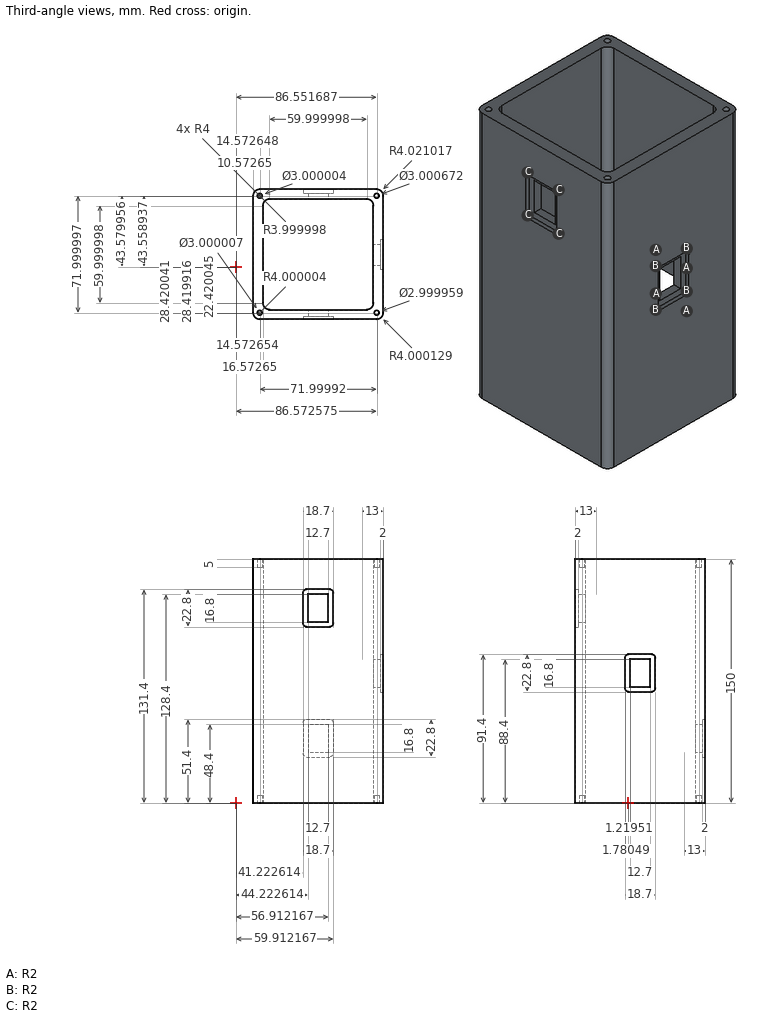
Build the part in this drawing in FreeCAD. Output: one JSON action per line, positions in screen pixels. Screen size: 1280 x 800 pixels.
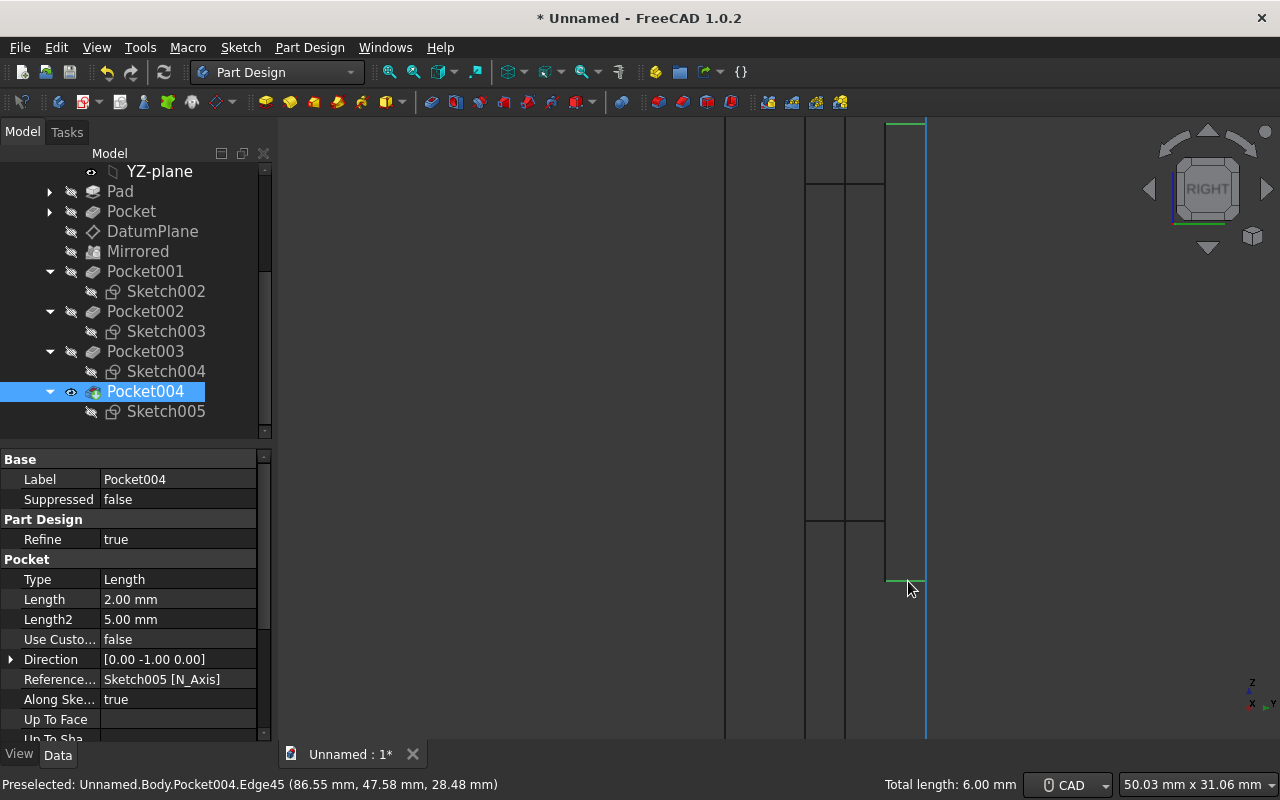
{"action": "left_click", "coordinate": [390, 72]}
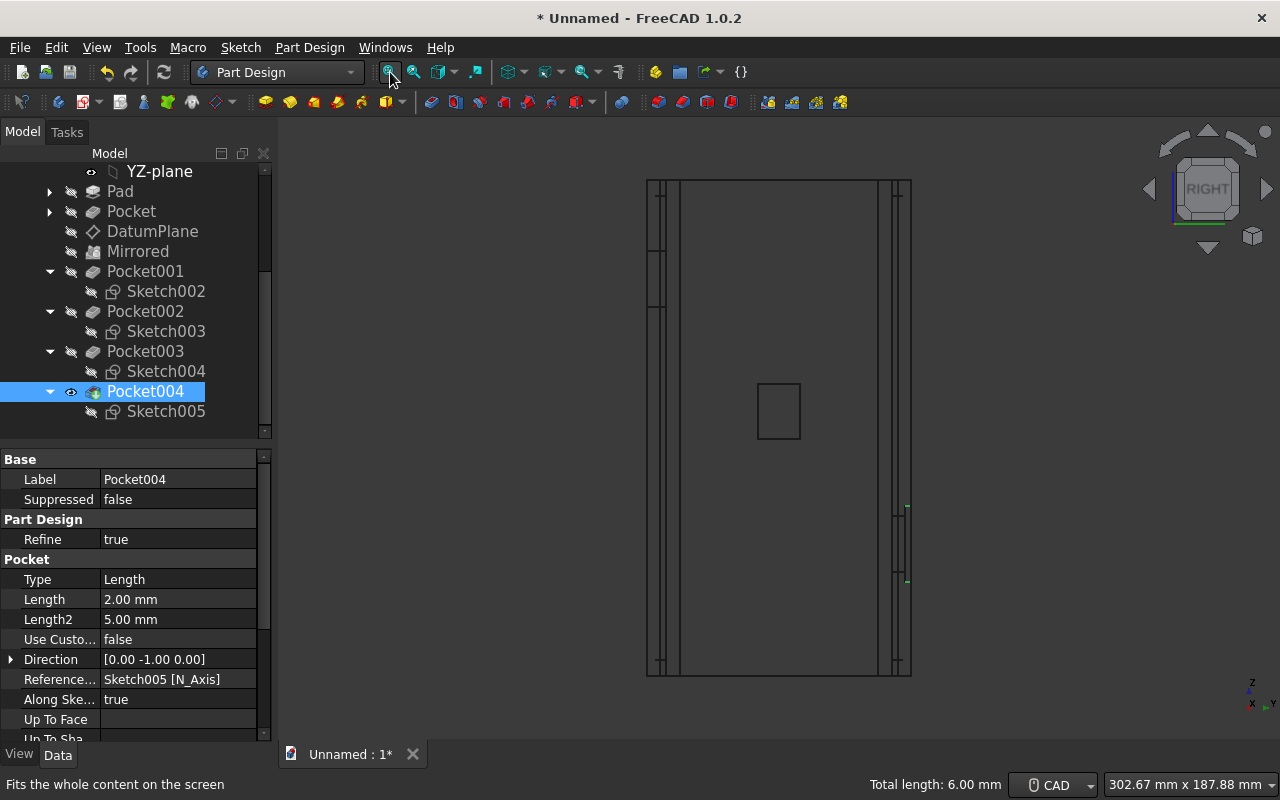
{"action": "key", "text": "5"}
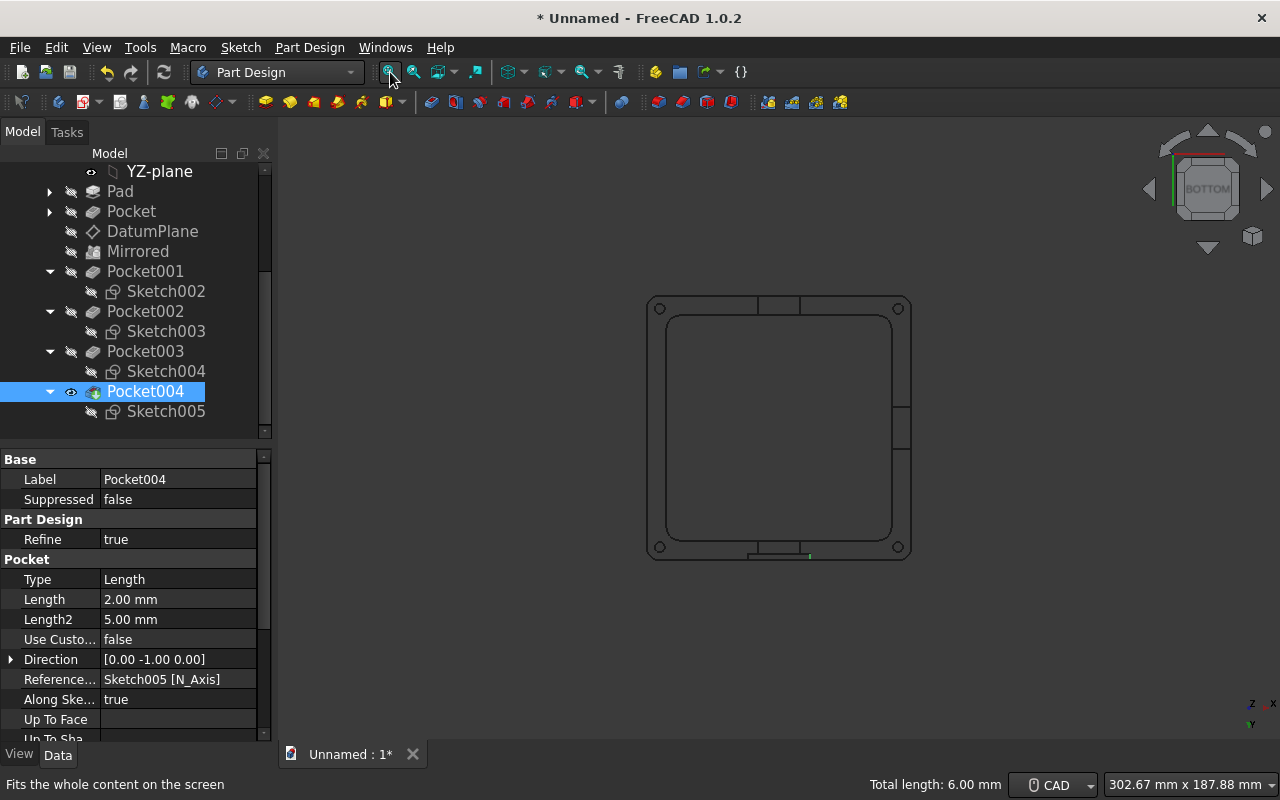
{"action": "left_click", "coordinate": [390, 72]}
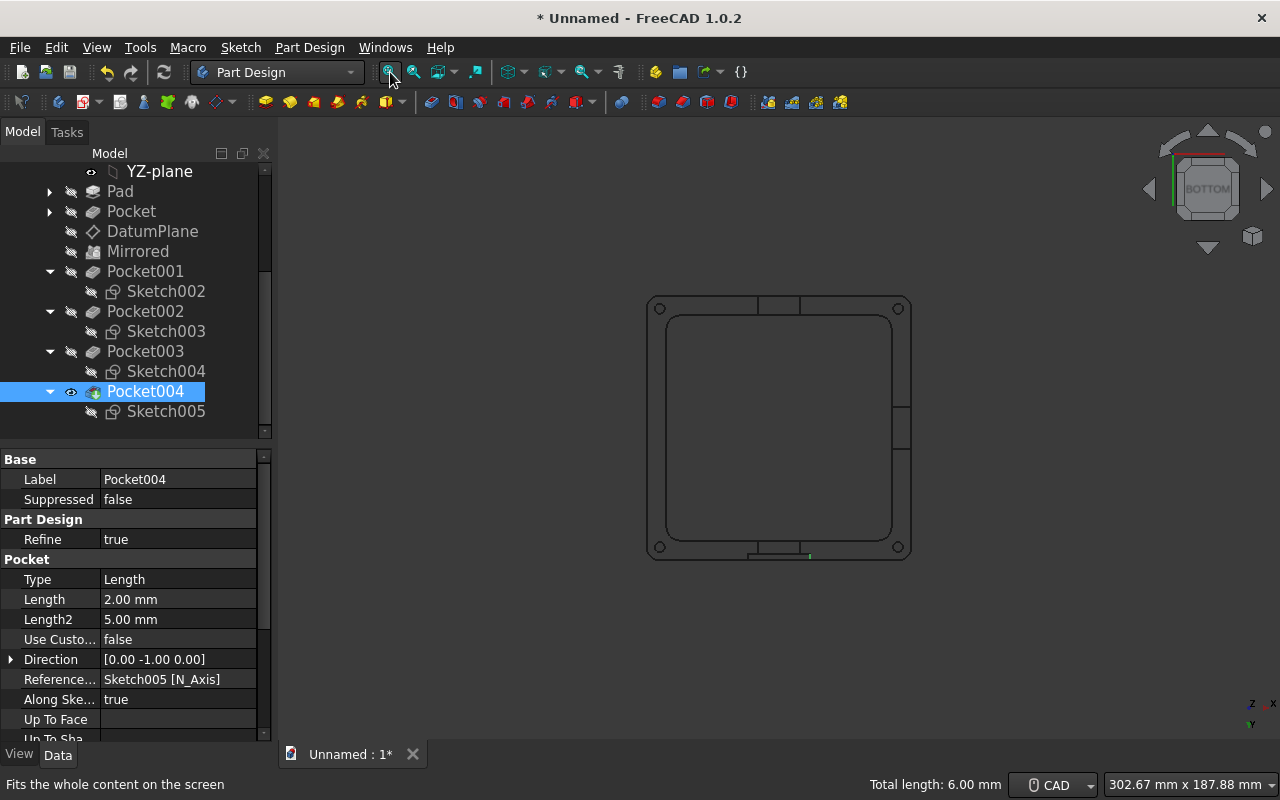
{"action": "scroll", "coordinate": [748, 556], "scroll_direction": "up", "scroll_amount": 9}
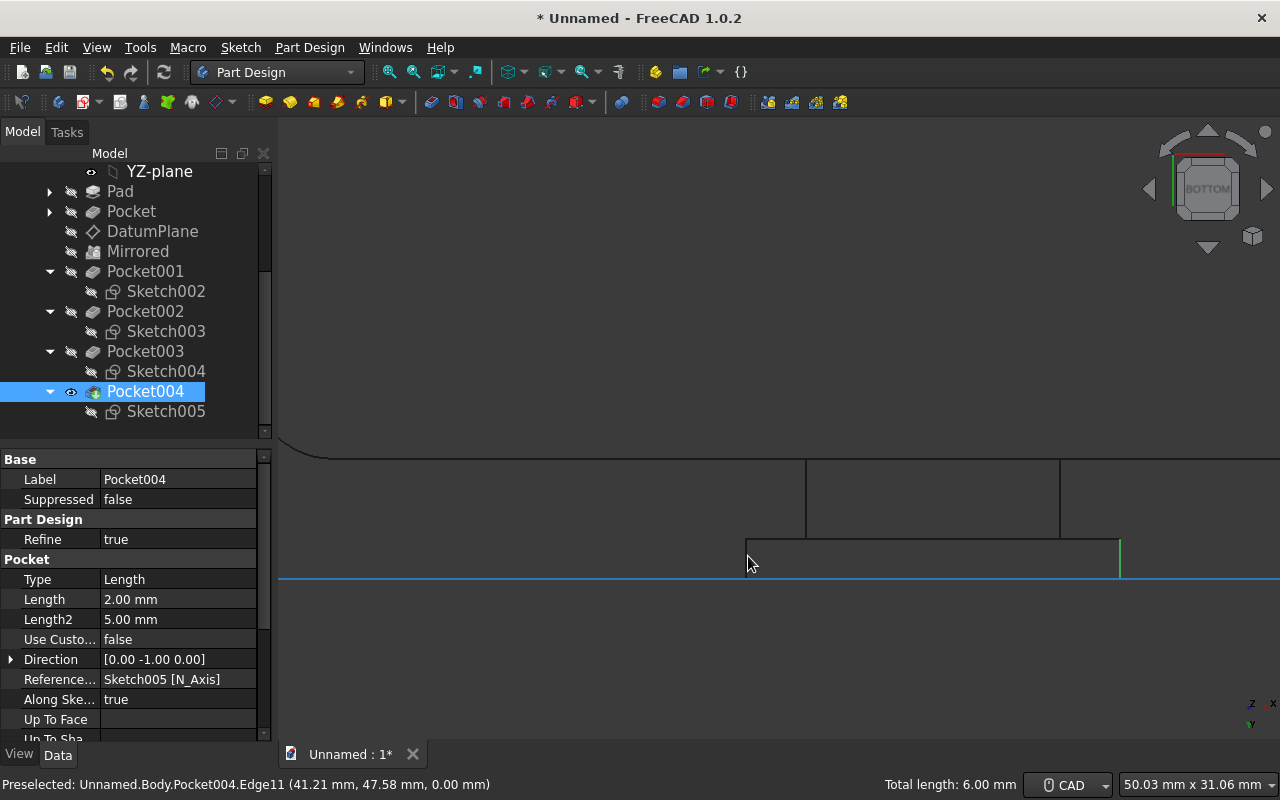
{"action": "left_click", "coordinate": [746, 558], "text": "ctrl"}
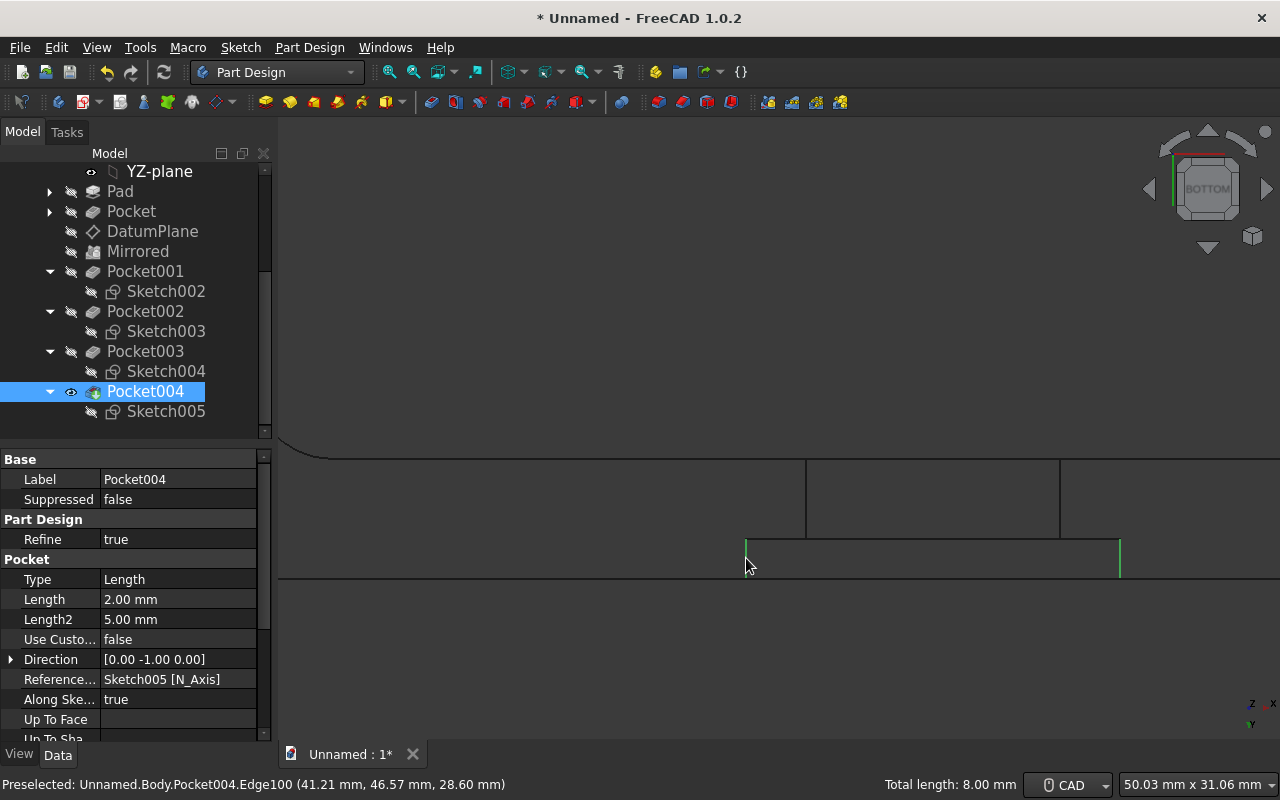
{"action": "key", "text": "v 1"}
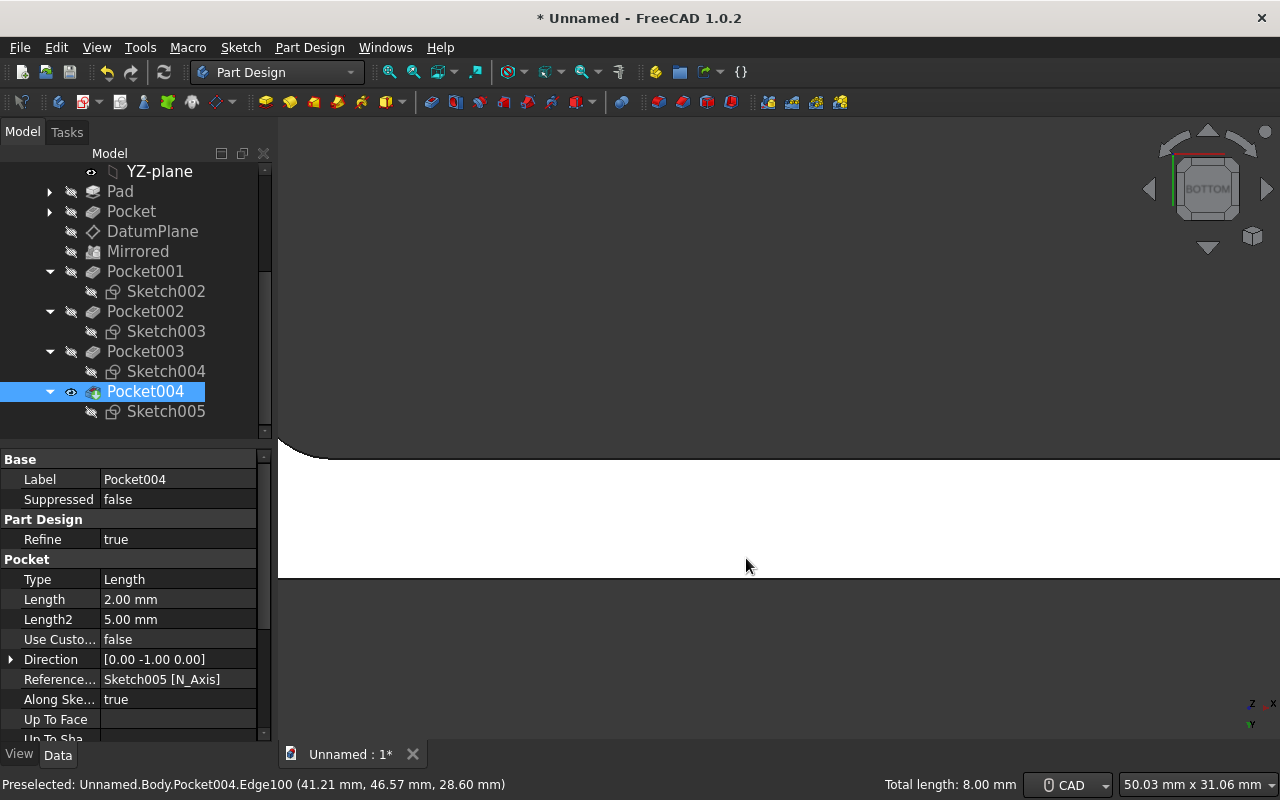
{"action": "left_click", "coordinate": [660, 102]}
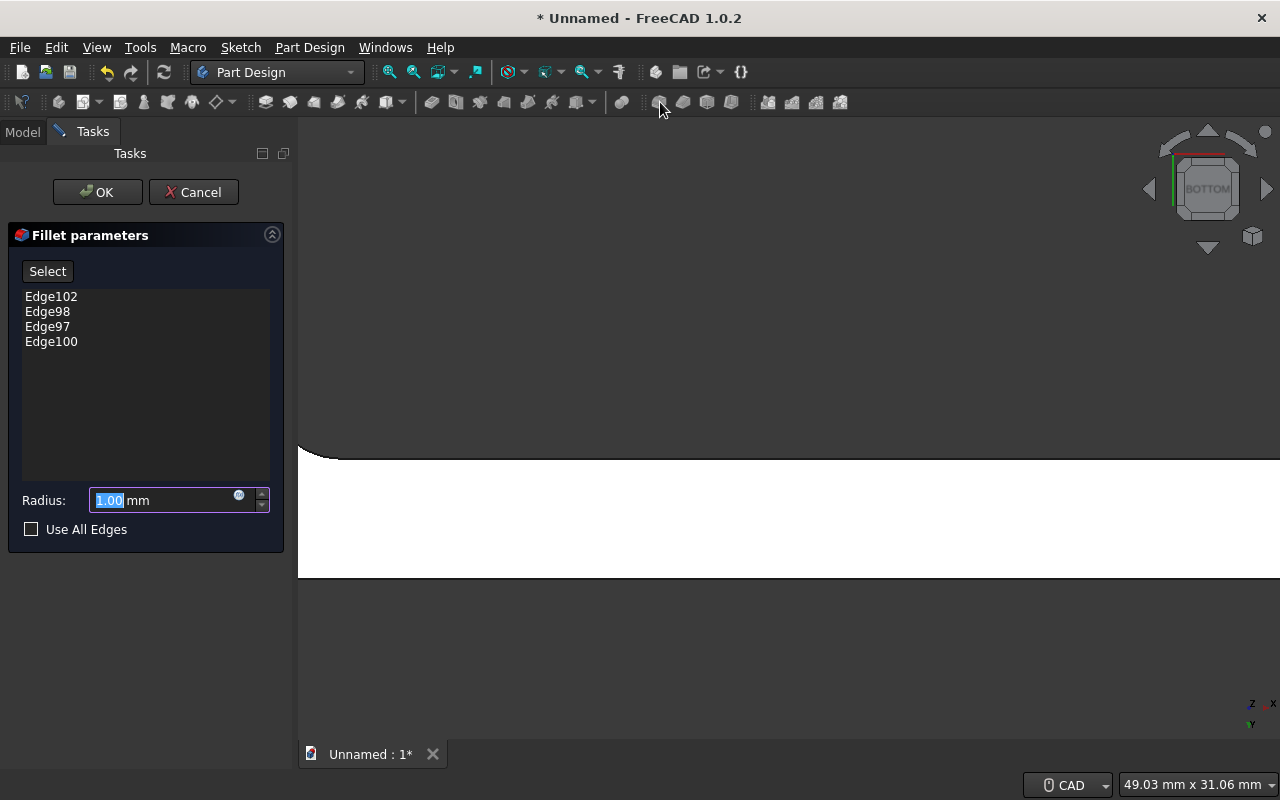
{"action": "type", "text": "2"}
{"action": "key", "text": "Tab"}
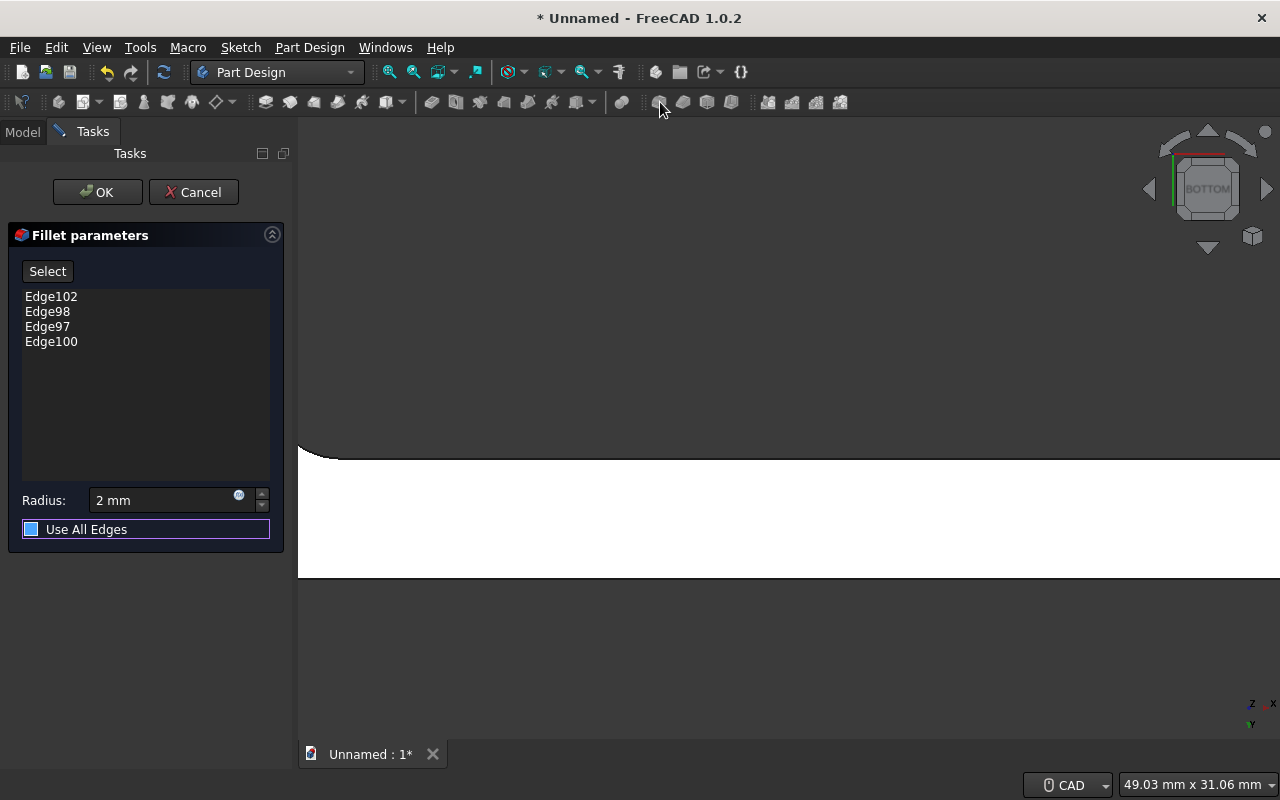
{"action": "left_click", "coordinate": [98, 192]}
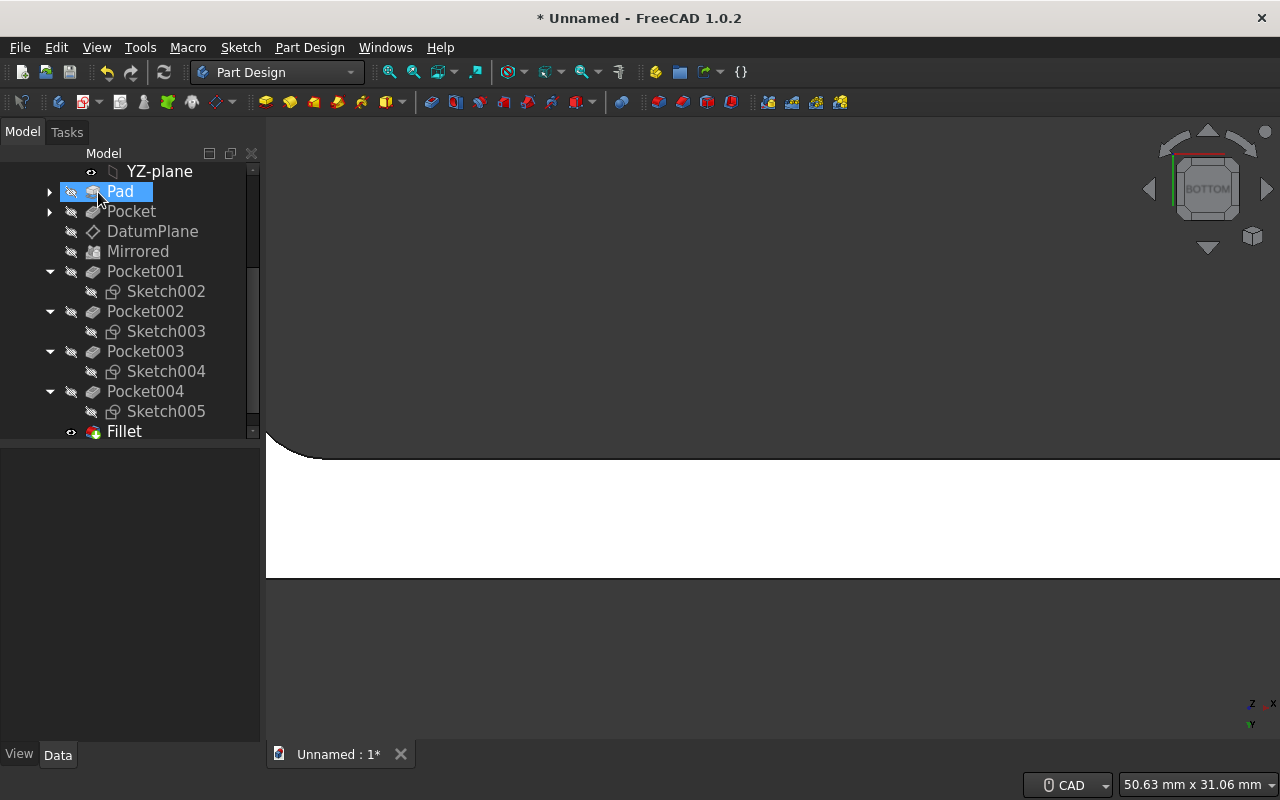
{"action": "left_click", "coordinate": [390, 72]}